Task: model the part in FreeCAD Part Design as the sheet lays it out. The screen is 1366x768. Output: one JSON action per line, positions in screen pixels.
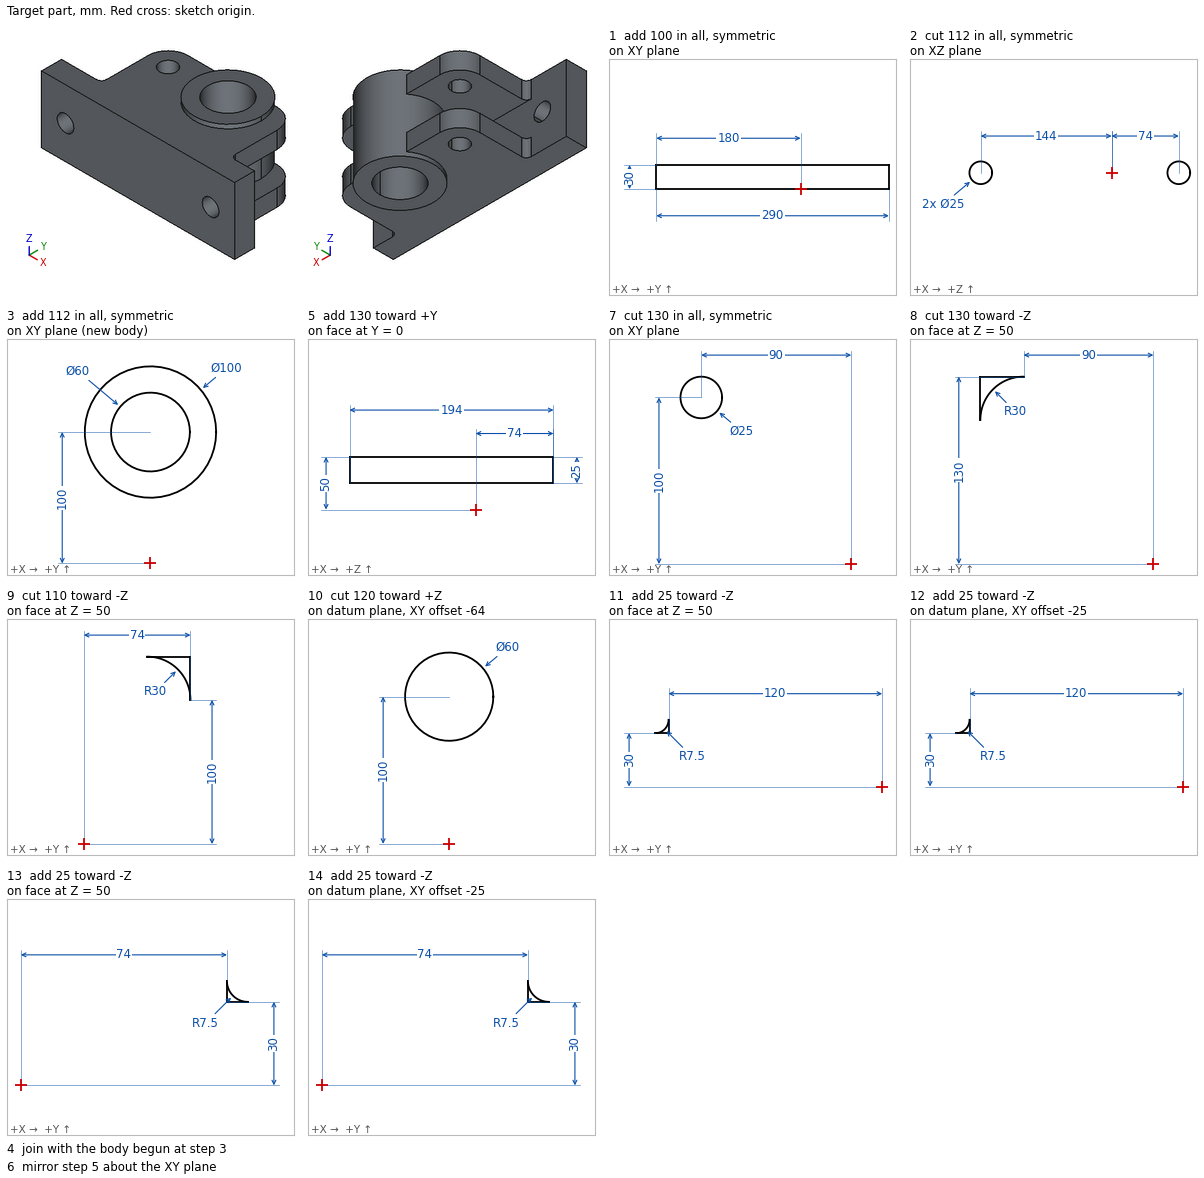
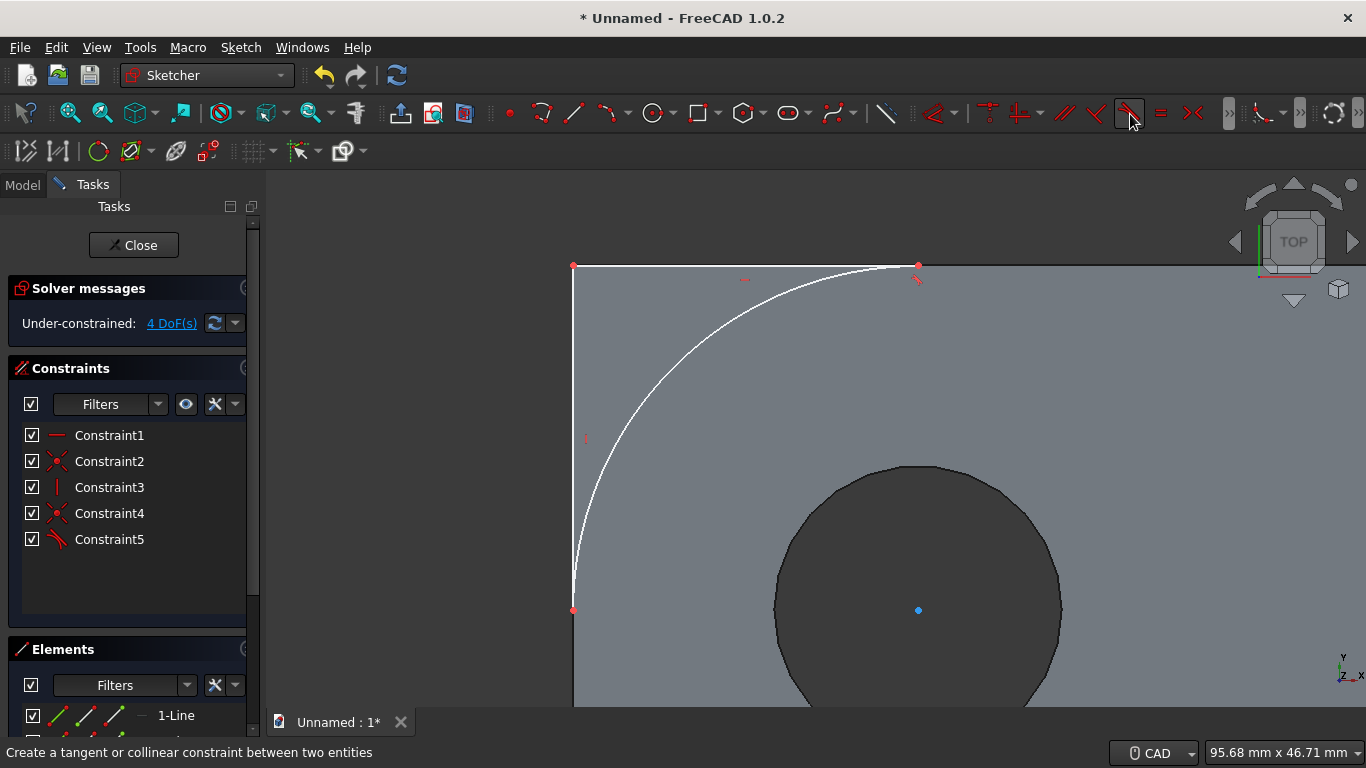
{"action": "left_click", "coordinate": [573, 369]}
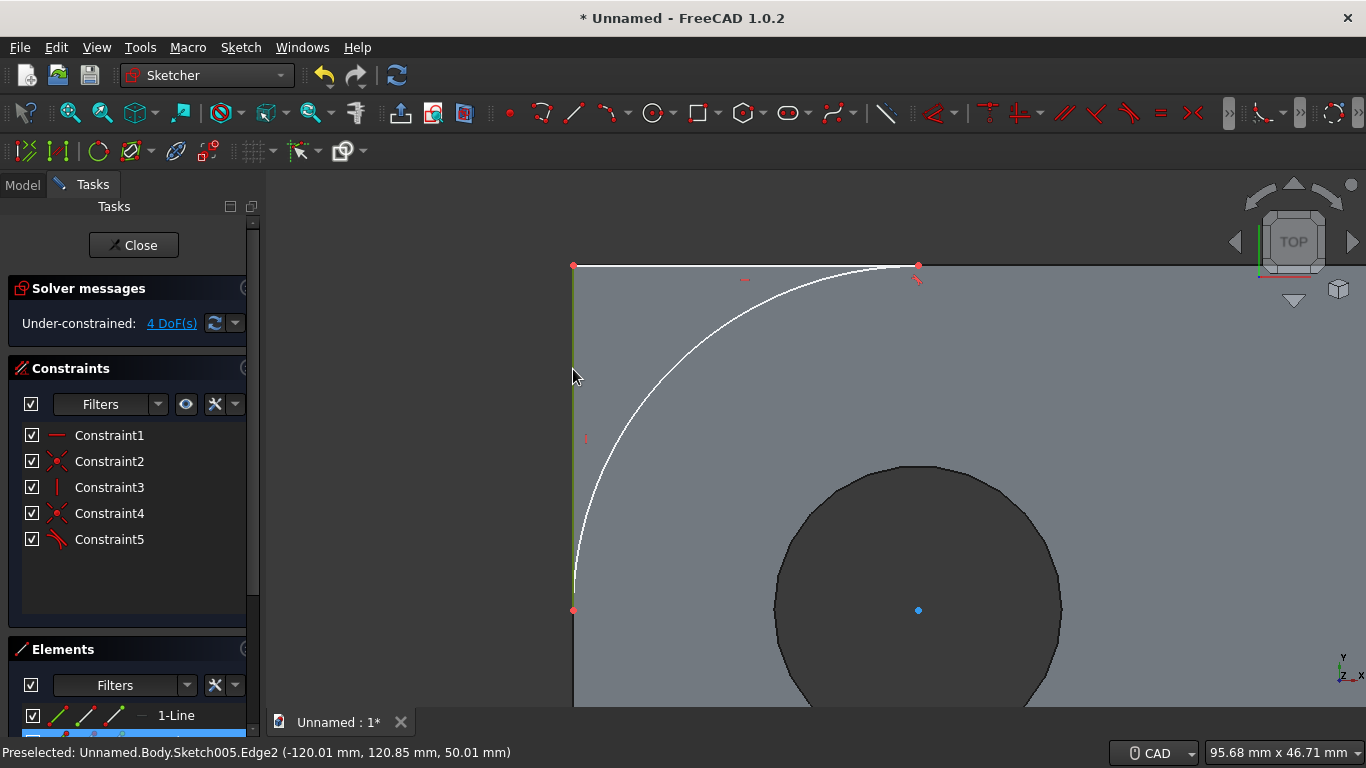
{"action": "left_click", "coordinate": [761, 304]}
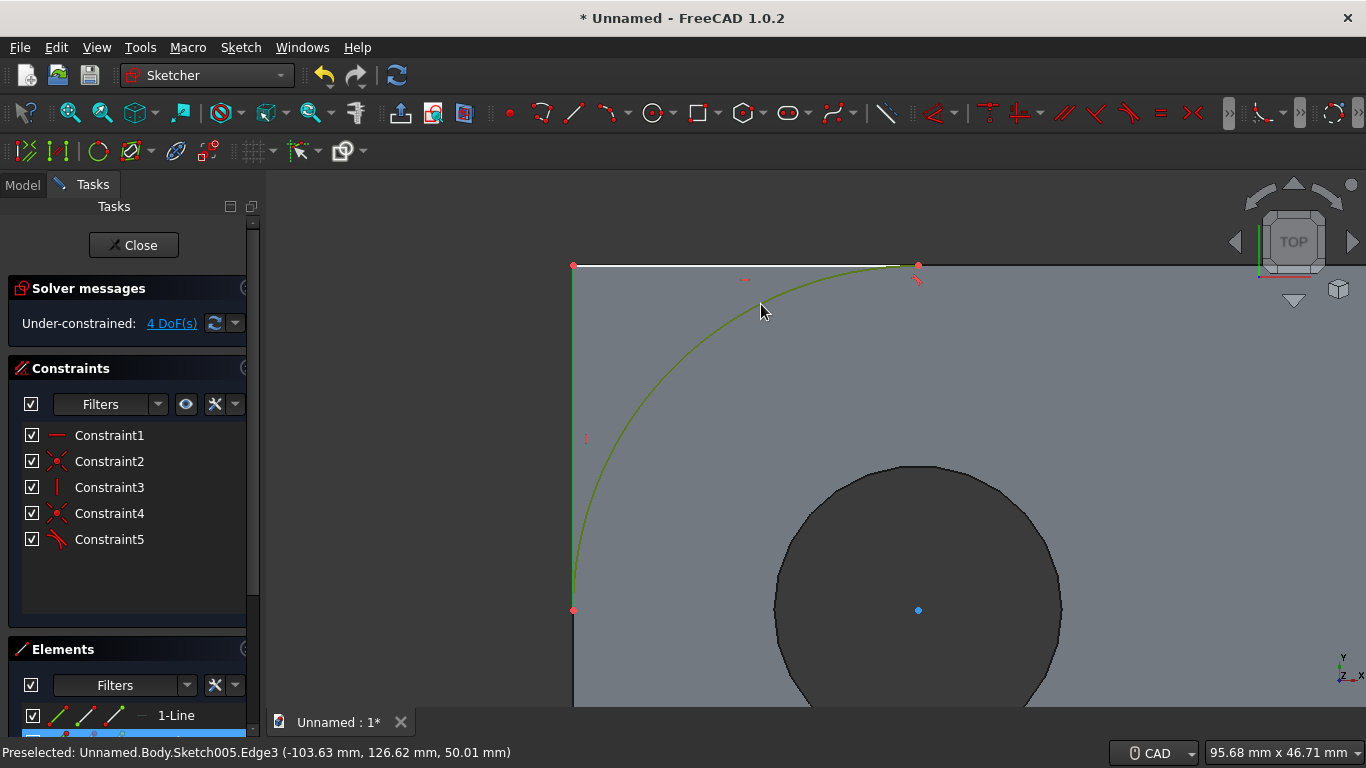
{"action": "left_click", "coordinate": [1130, 114]}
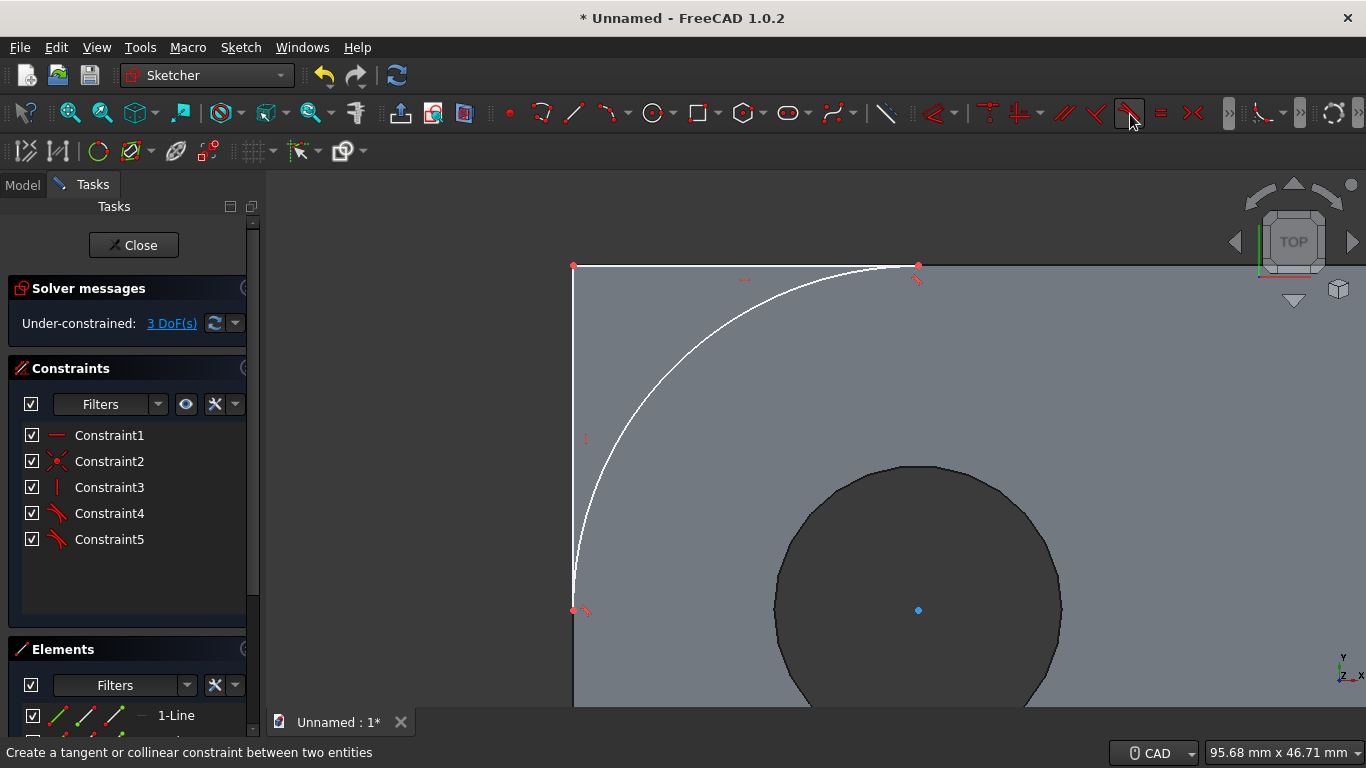
{"action": "left_click", "coordinate": [934, 114]}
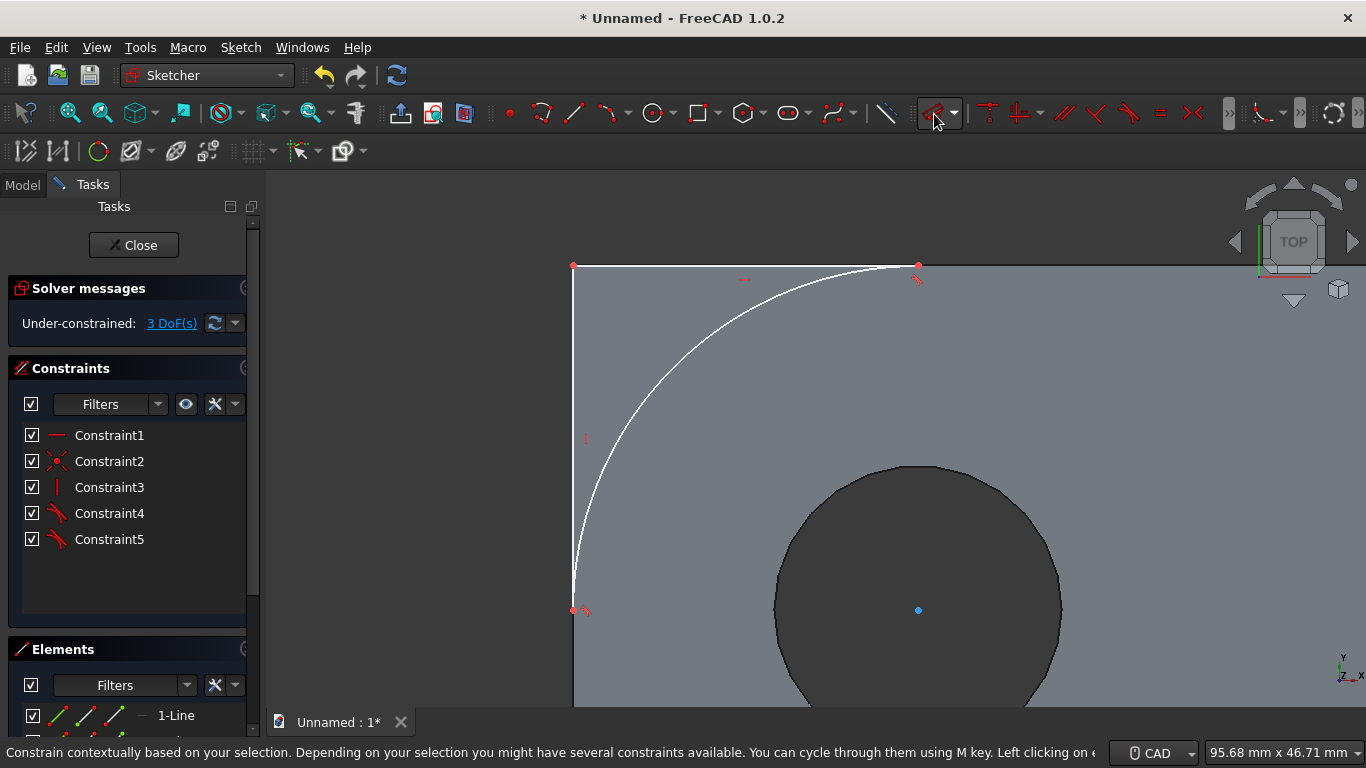
{"action": "left_click", "coordinate": [761, 304]}
{"action": "left_click", "coordinate": [928, 234]}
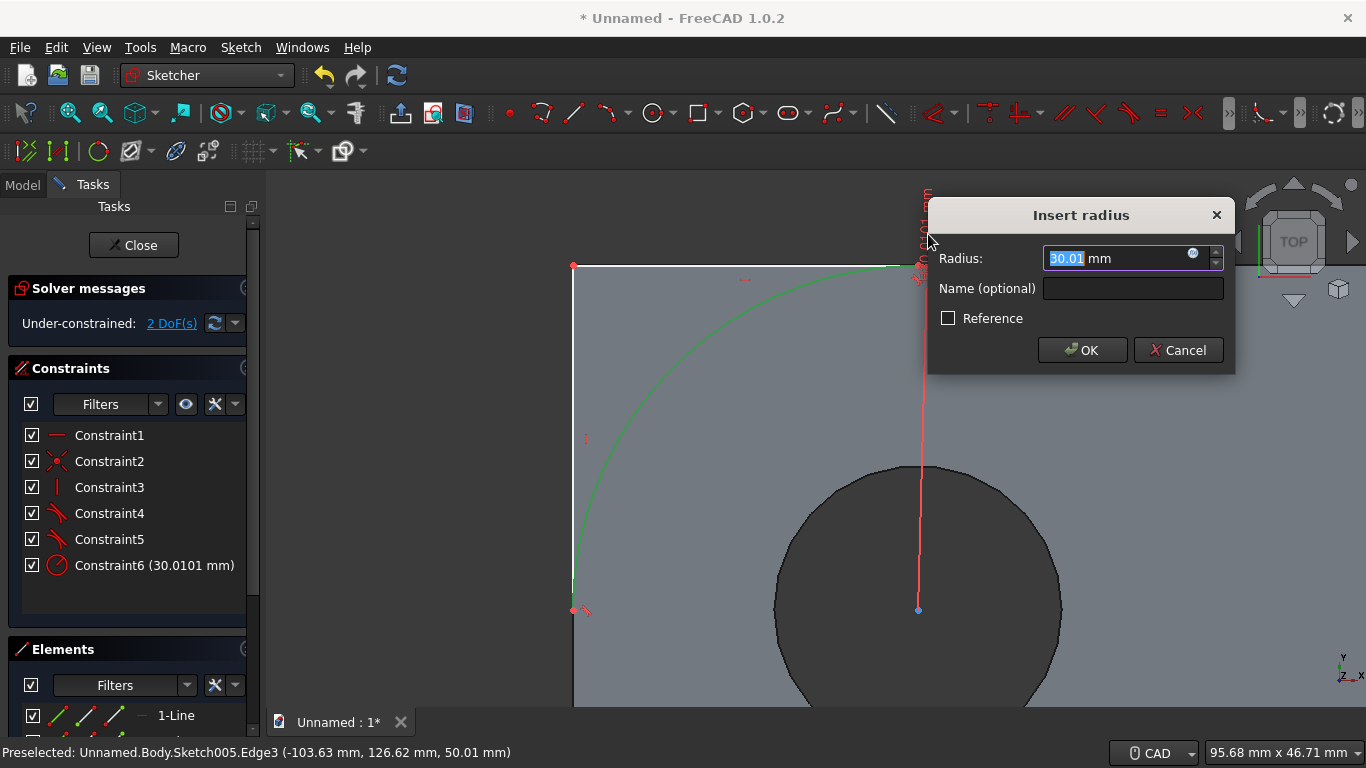
{"action": "type", "text": "30"}
{"action": "key", "text": "Return"}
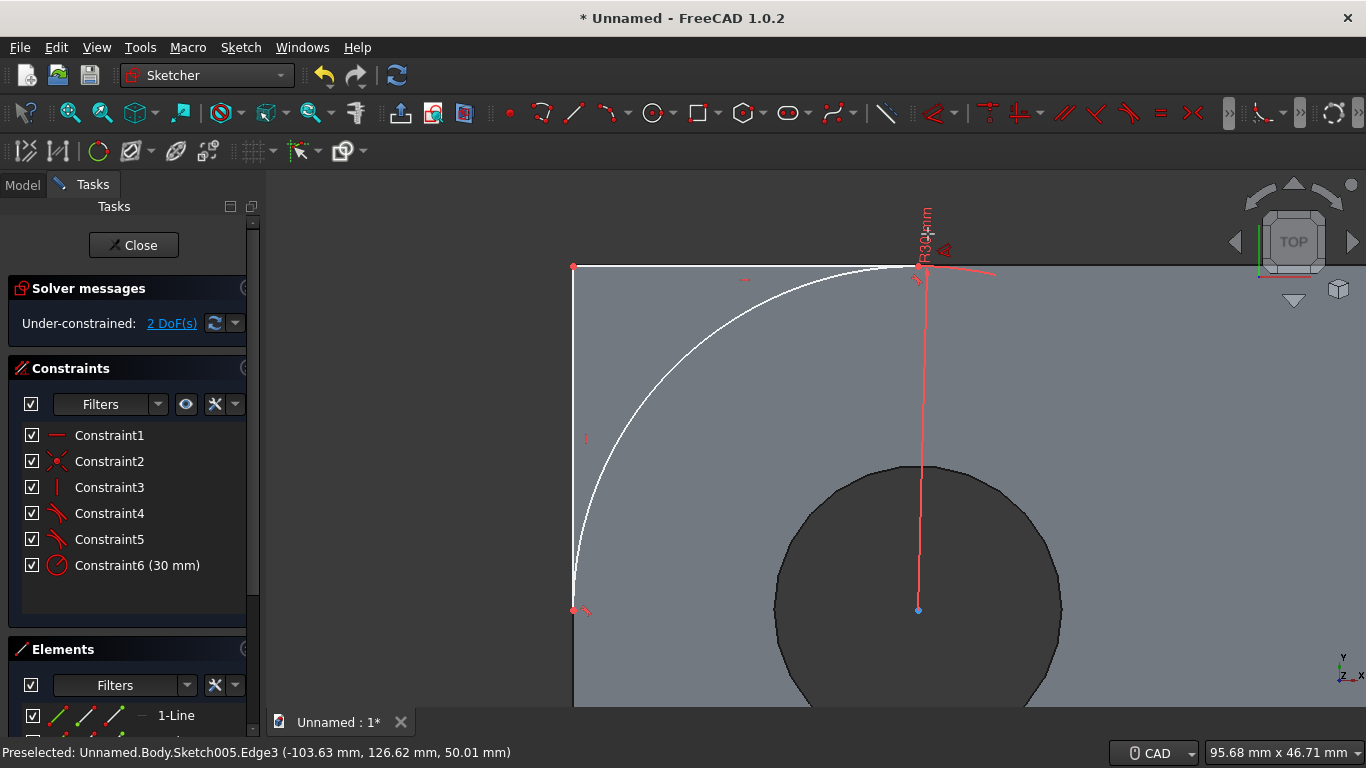
{"action": "left_click", "coordinate": [918, 266]}
{"action": "left_click", "coordinate": [1059, 232]}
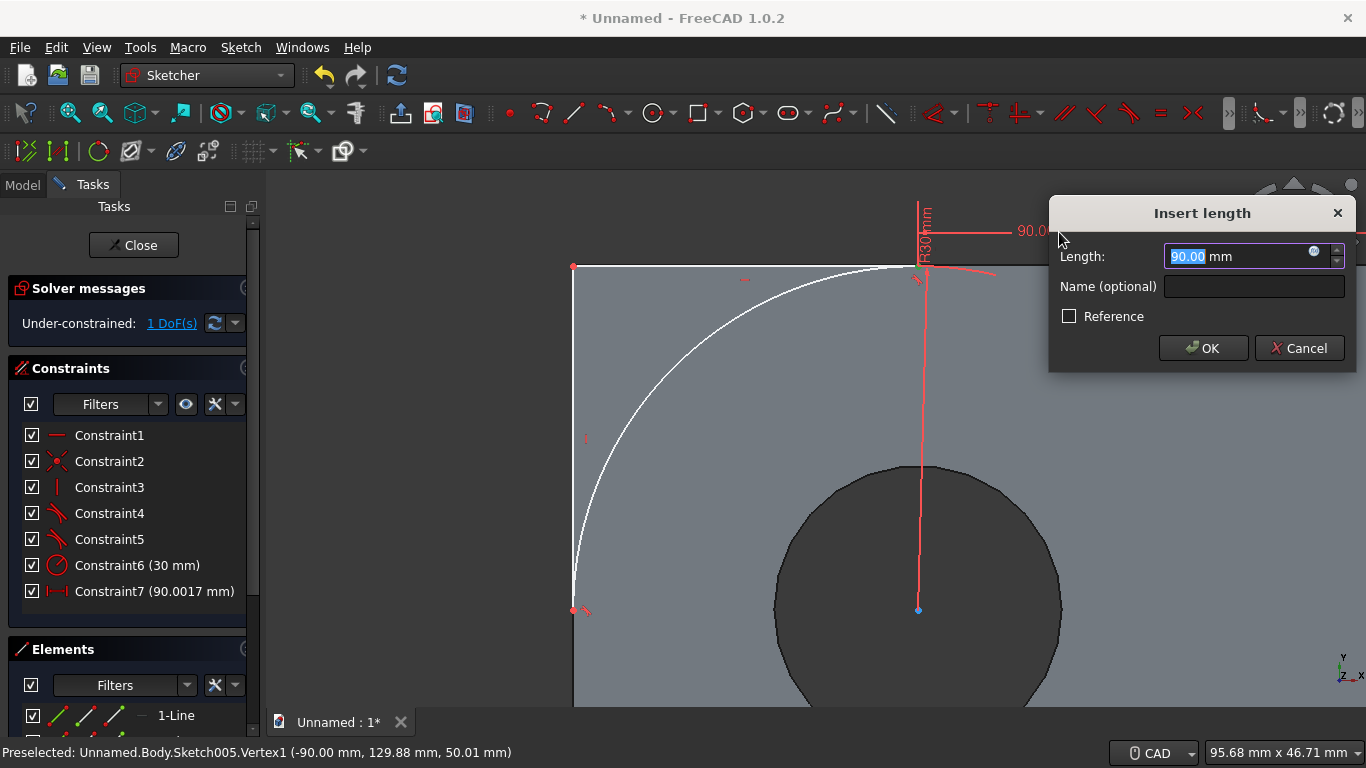
{"action": "type", "text": "90"}
{"action": "key", "text": "Return"}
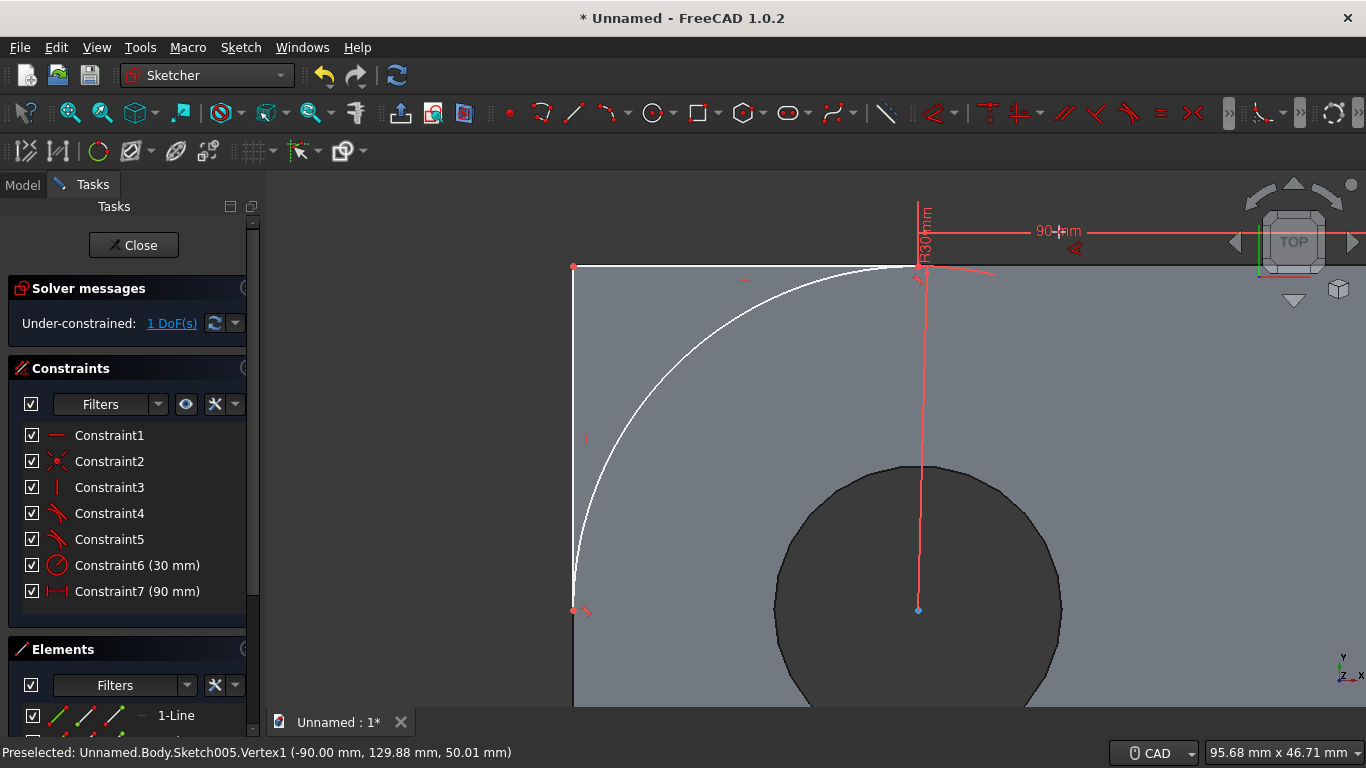
{"action": "left_click", "coordinate": [918, 266]}
{"action": "left_click", "coordinate": [884, 473]}